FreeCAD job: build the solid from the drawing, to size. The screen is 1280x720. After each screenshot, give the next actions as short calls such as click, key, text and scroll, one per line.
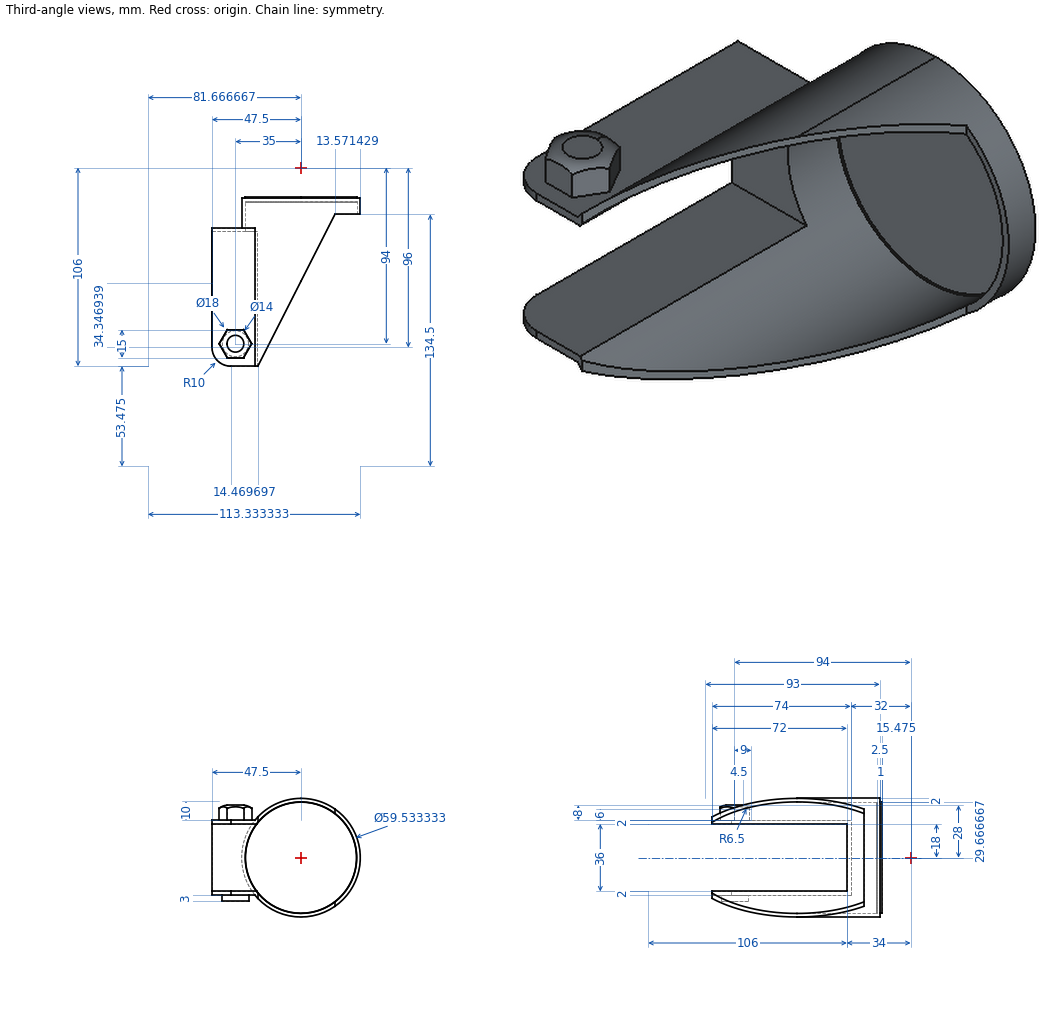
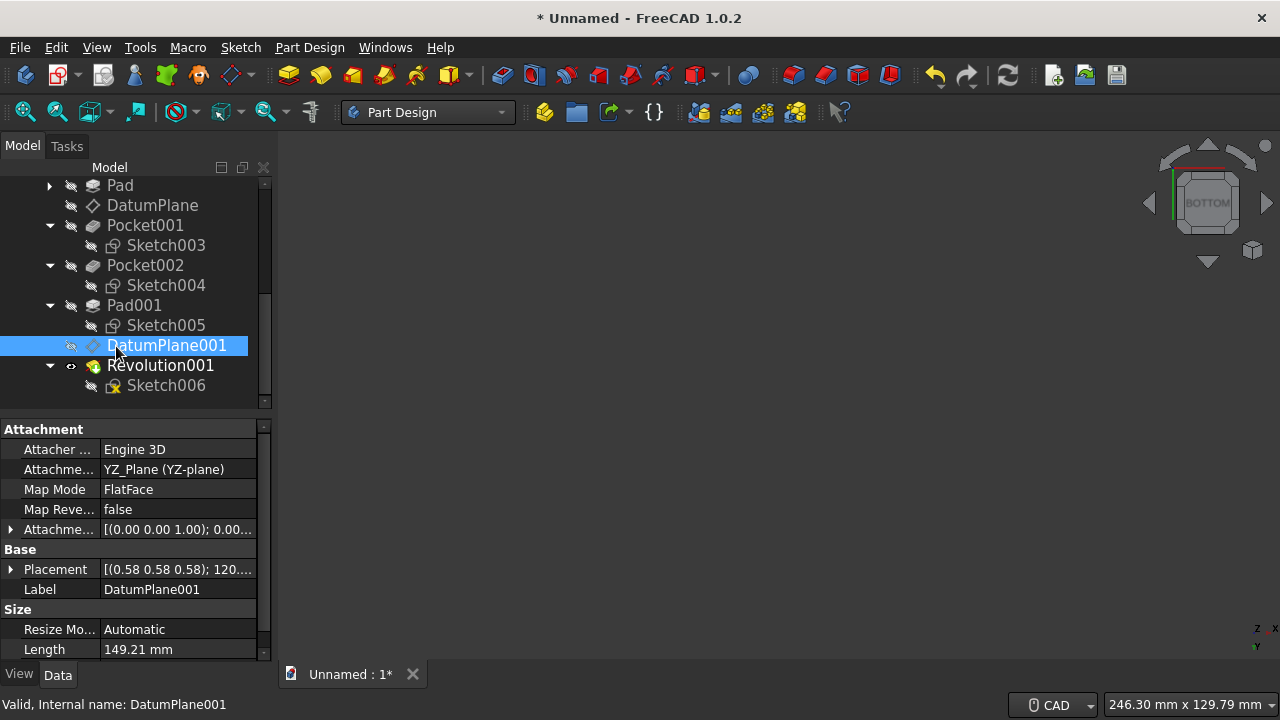
click(26, 112)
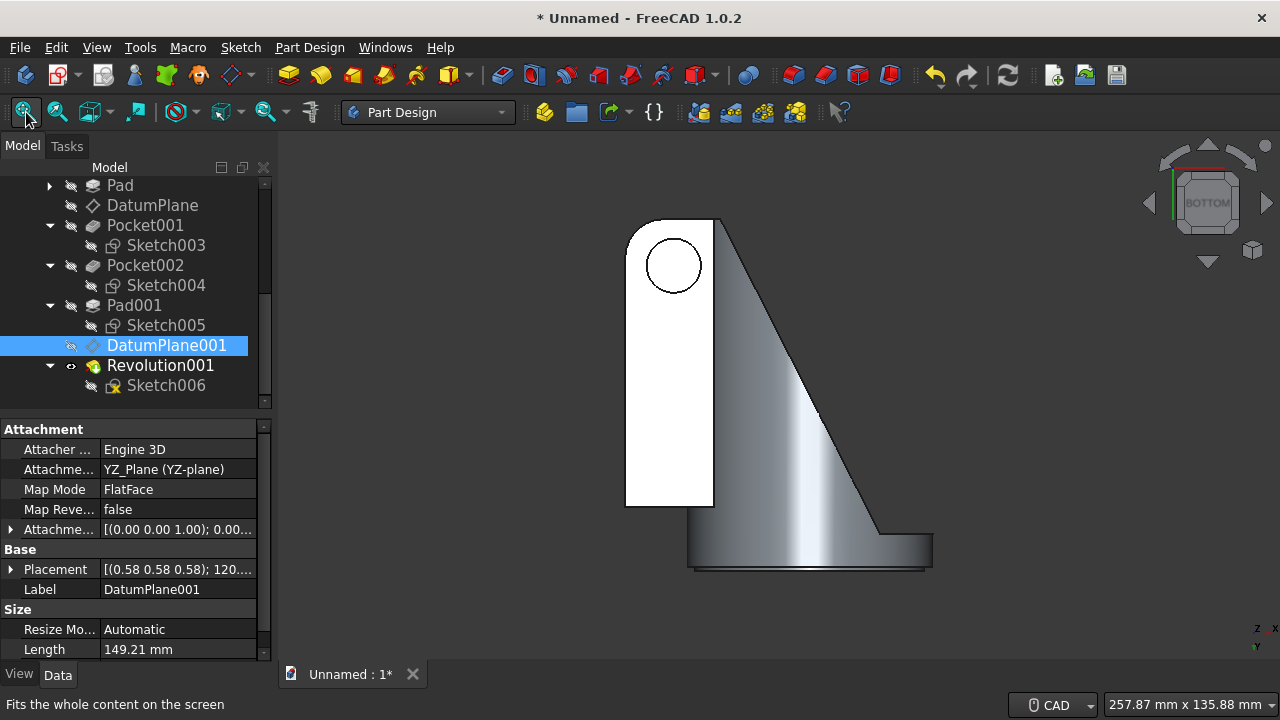
key(0)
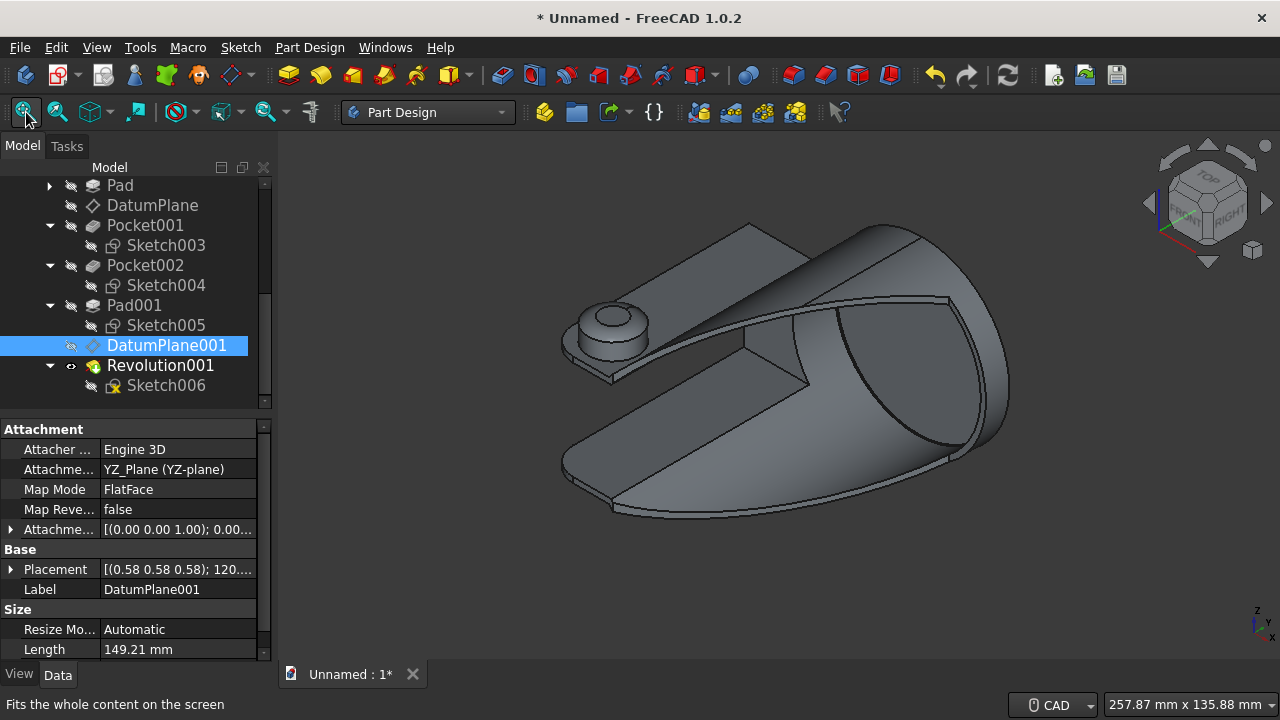
click(737, 266)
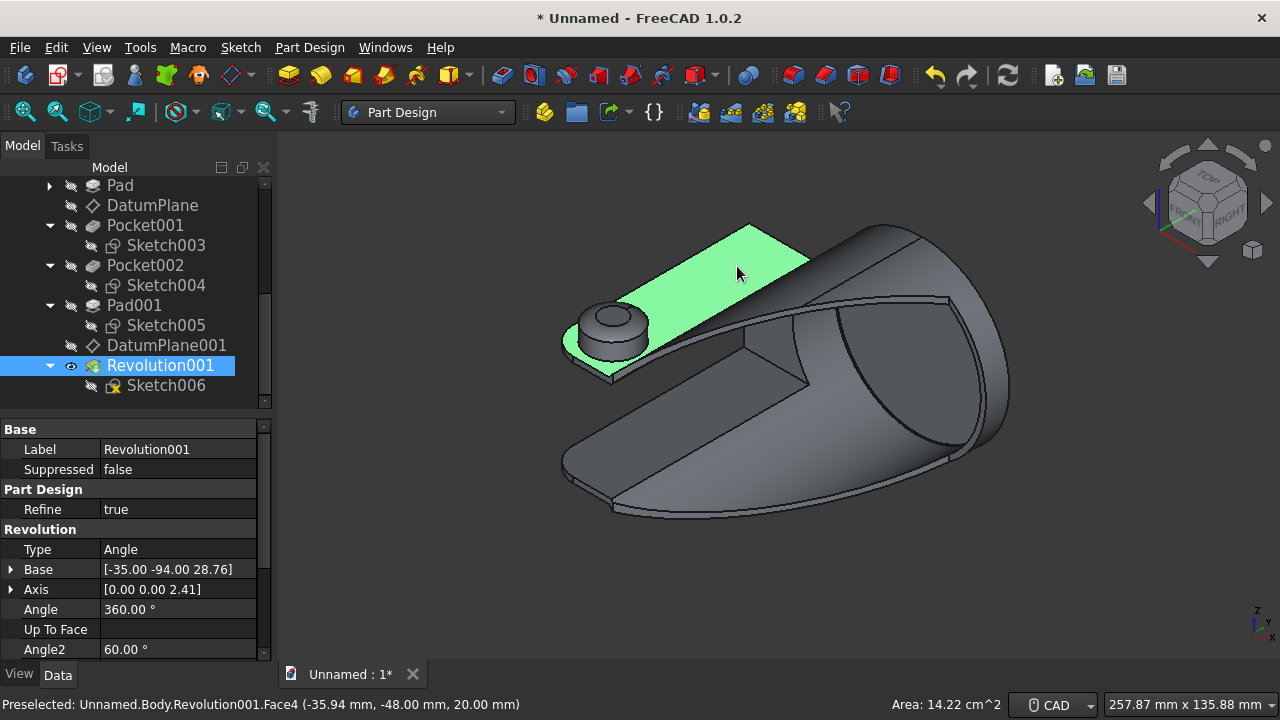
click(58, 76)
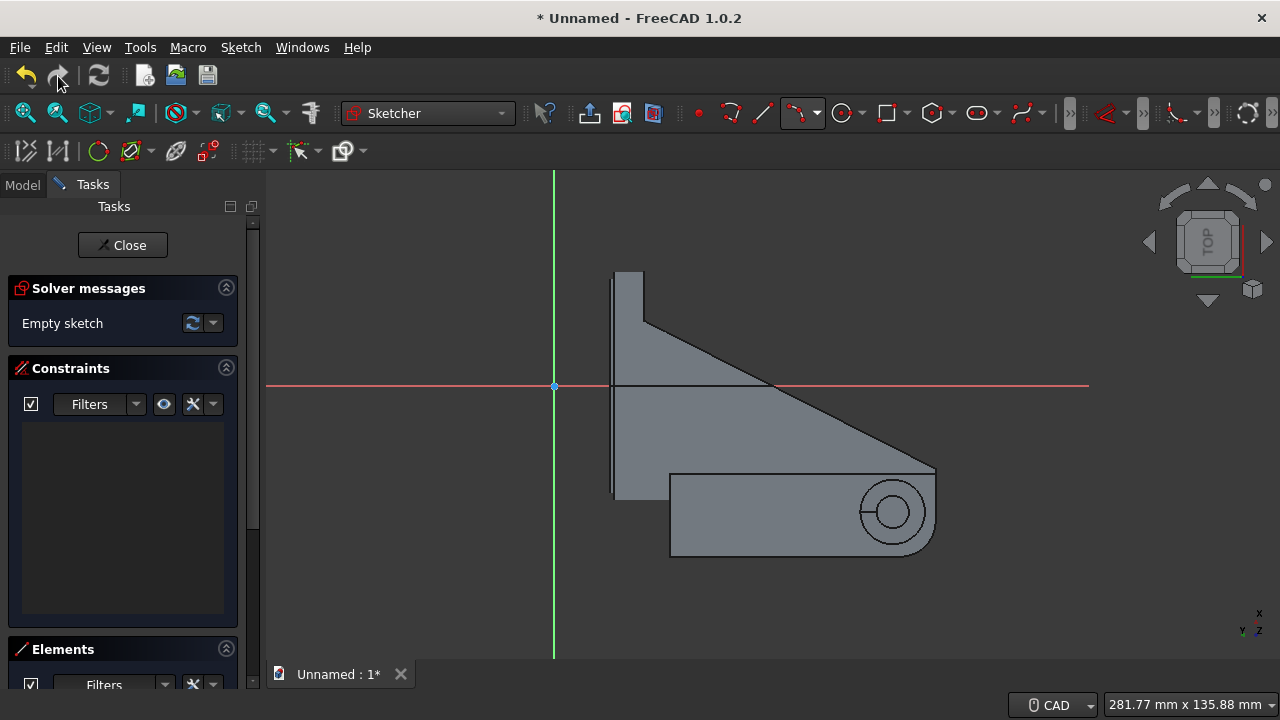
scroll(940, 537, up, 8)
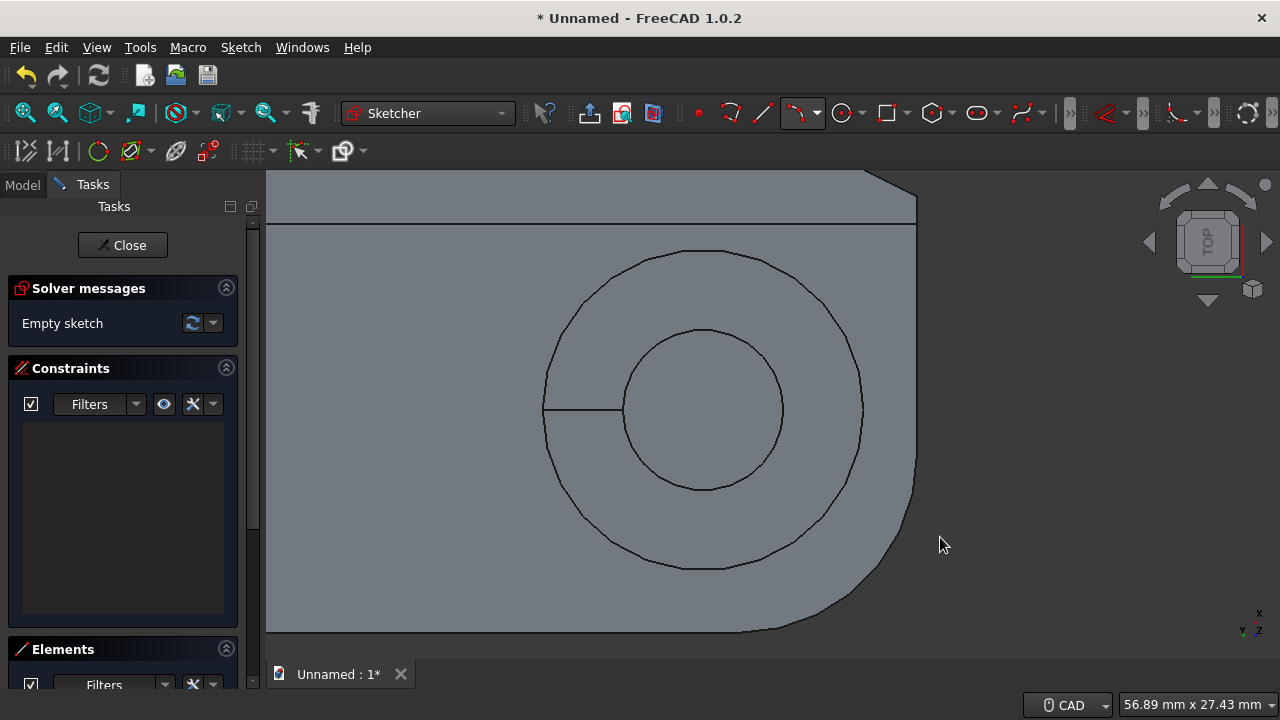
click(932, 114)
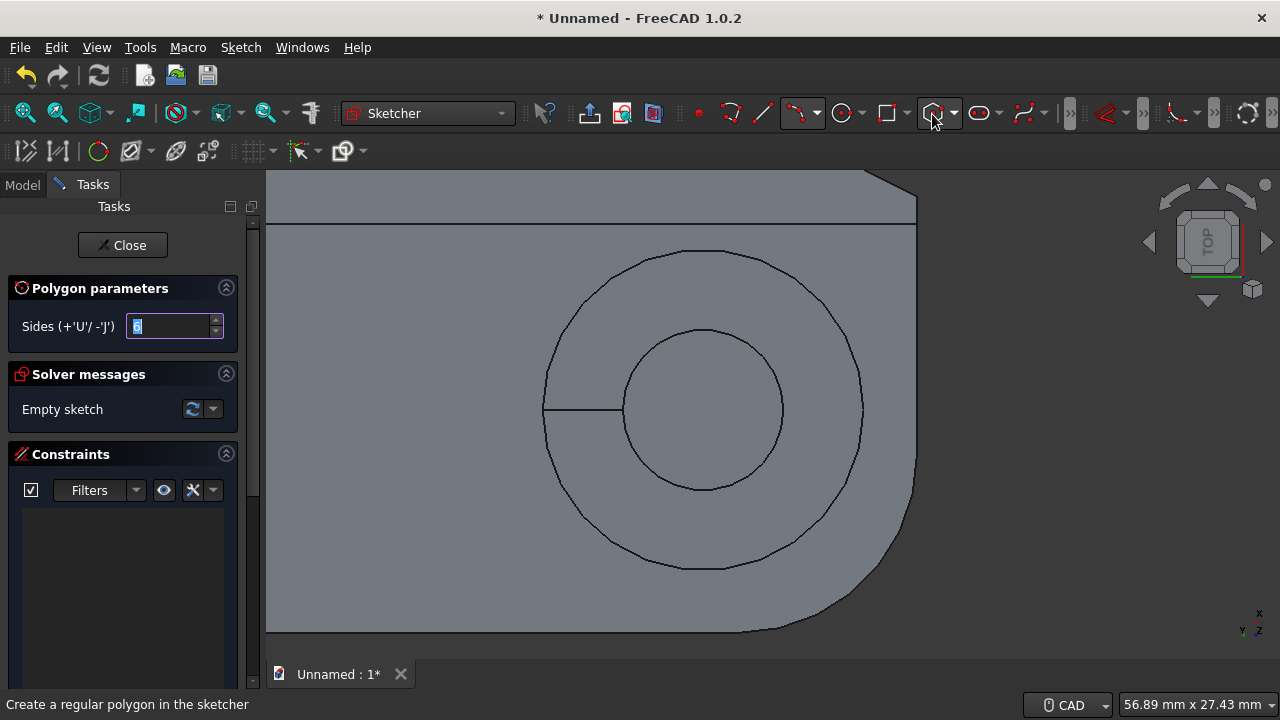
click(703, 410)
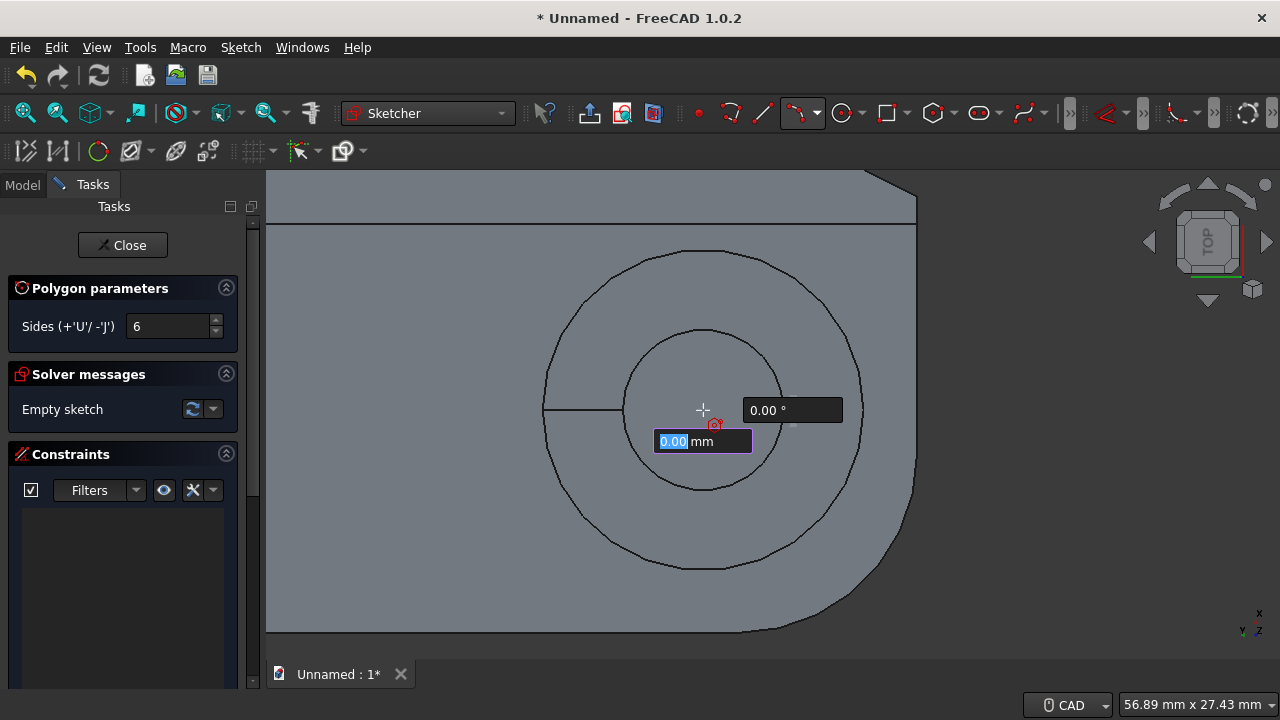
click(703, 564)
key(Escape)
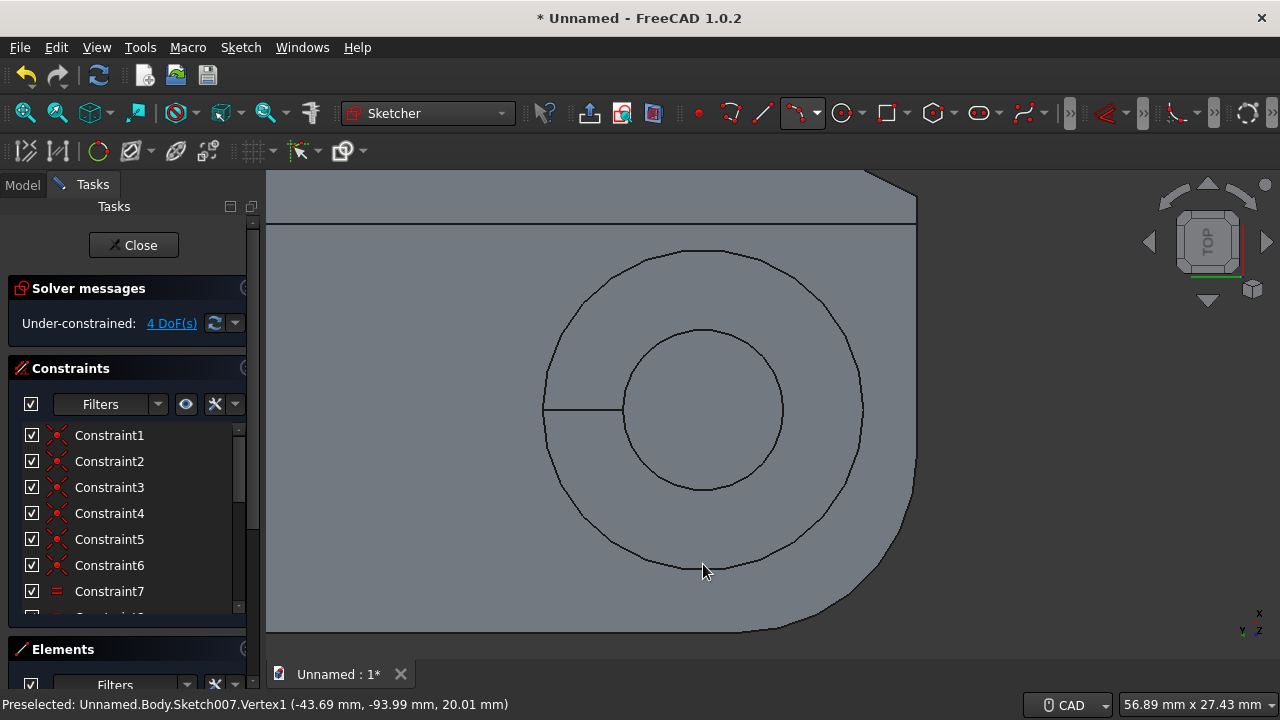
click(842, 114)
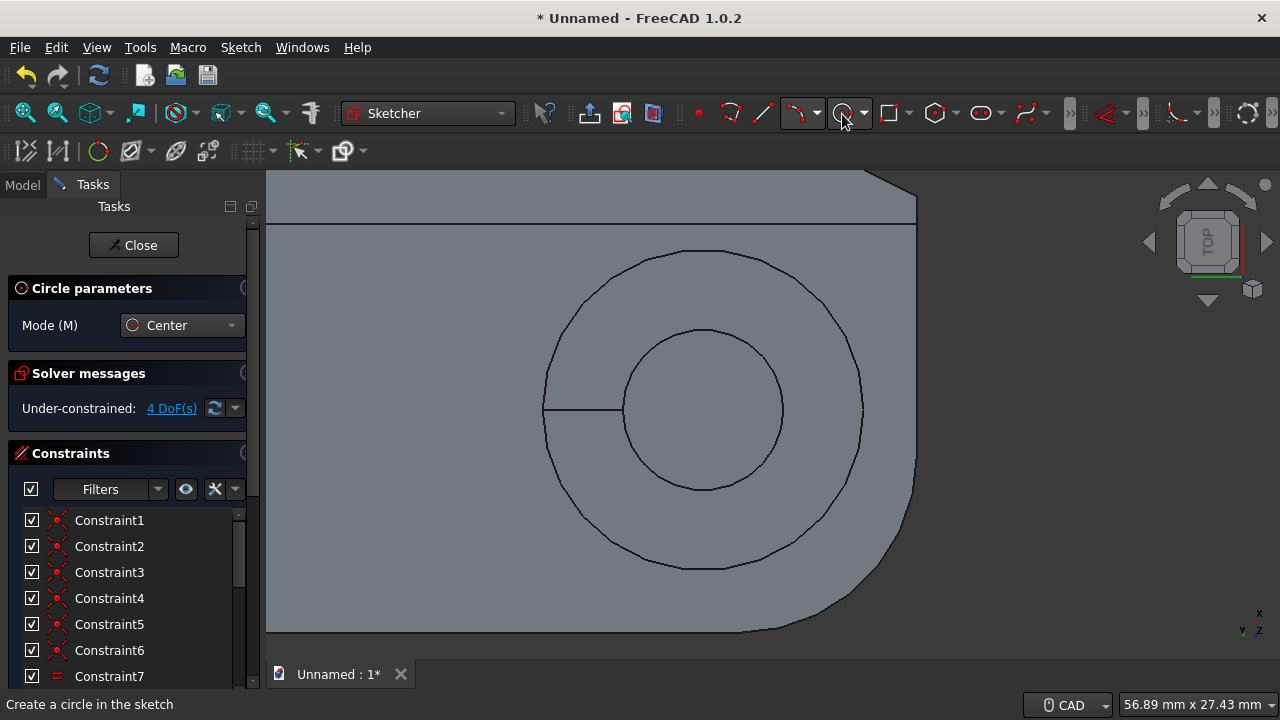
click(703, 411)
click(817, 297)
key(Escape)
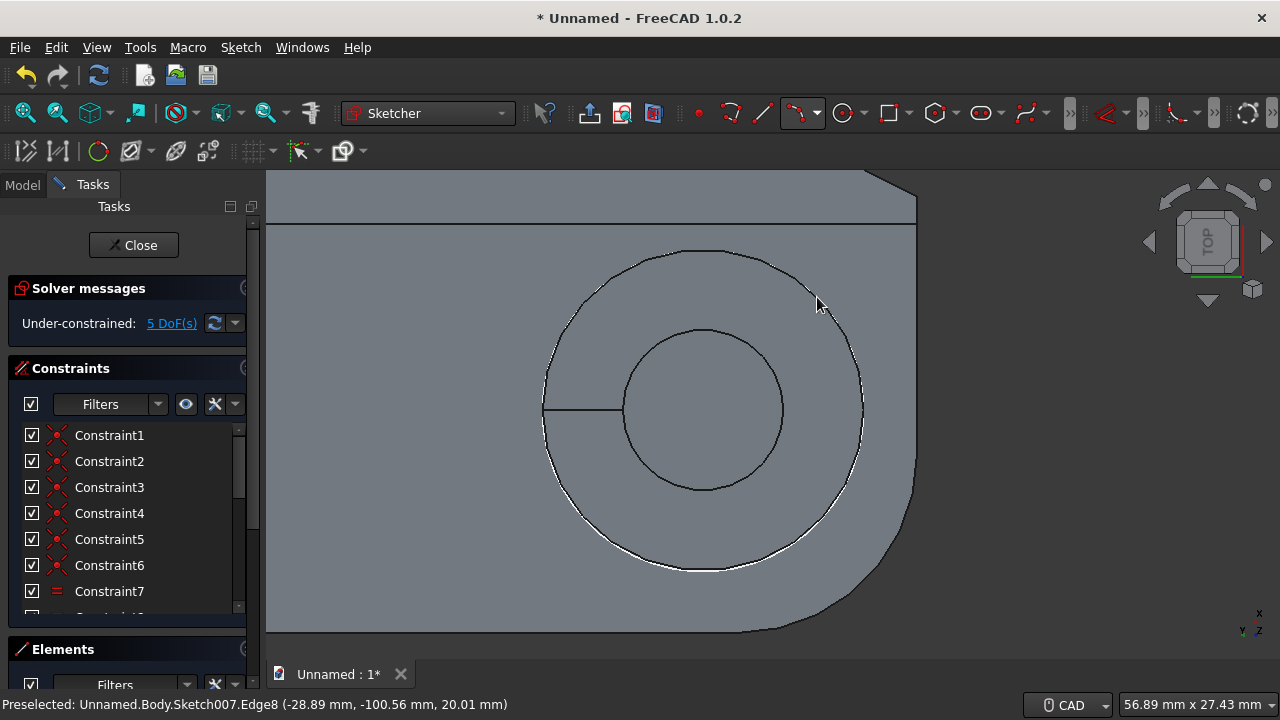
click(836, 442)